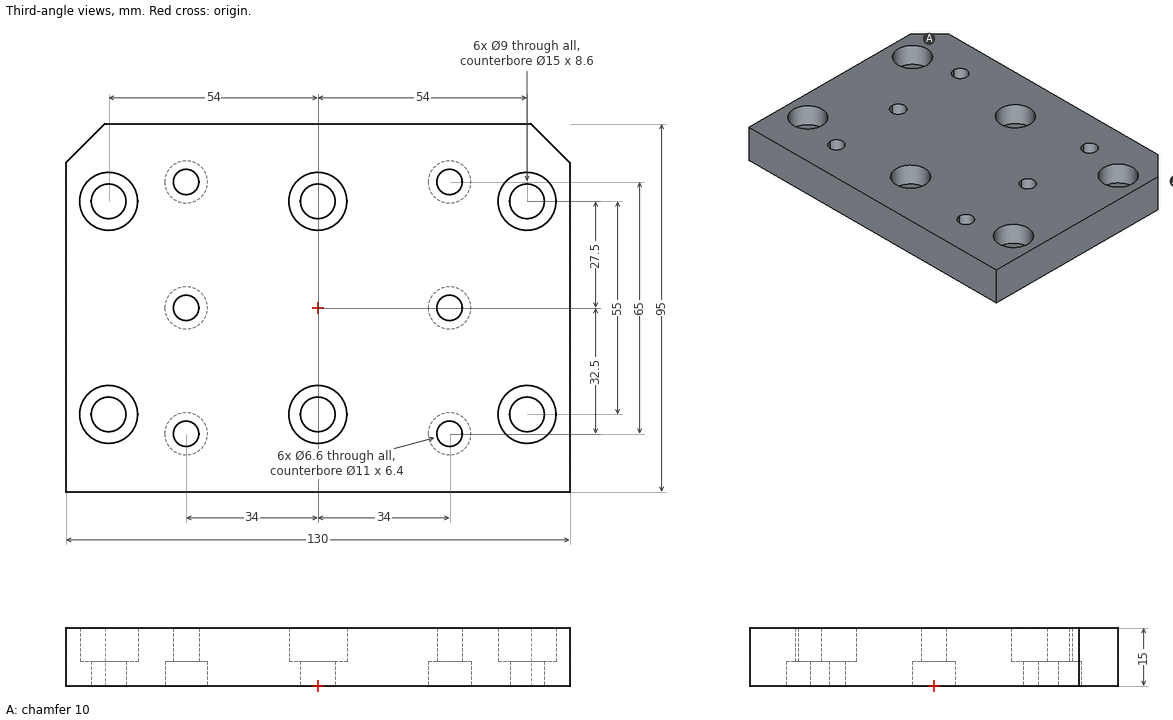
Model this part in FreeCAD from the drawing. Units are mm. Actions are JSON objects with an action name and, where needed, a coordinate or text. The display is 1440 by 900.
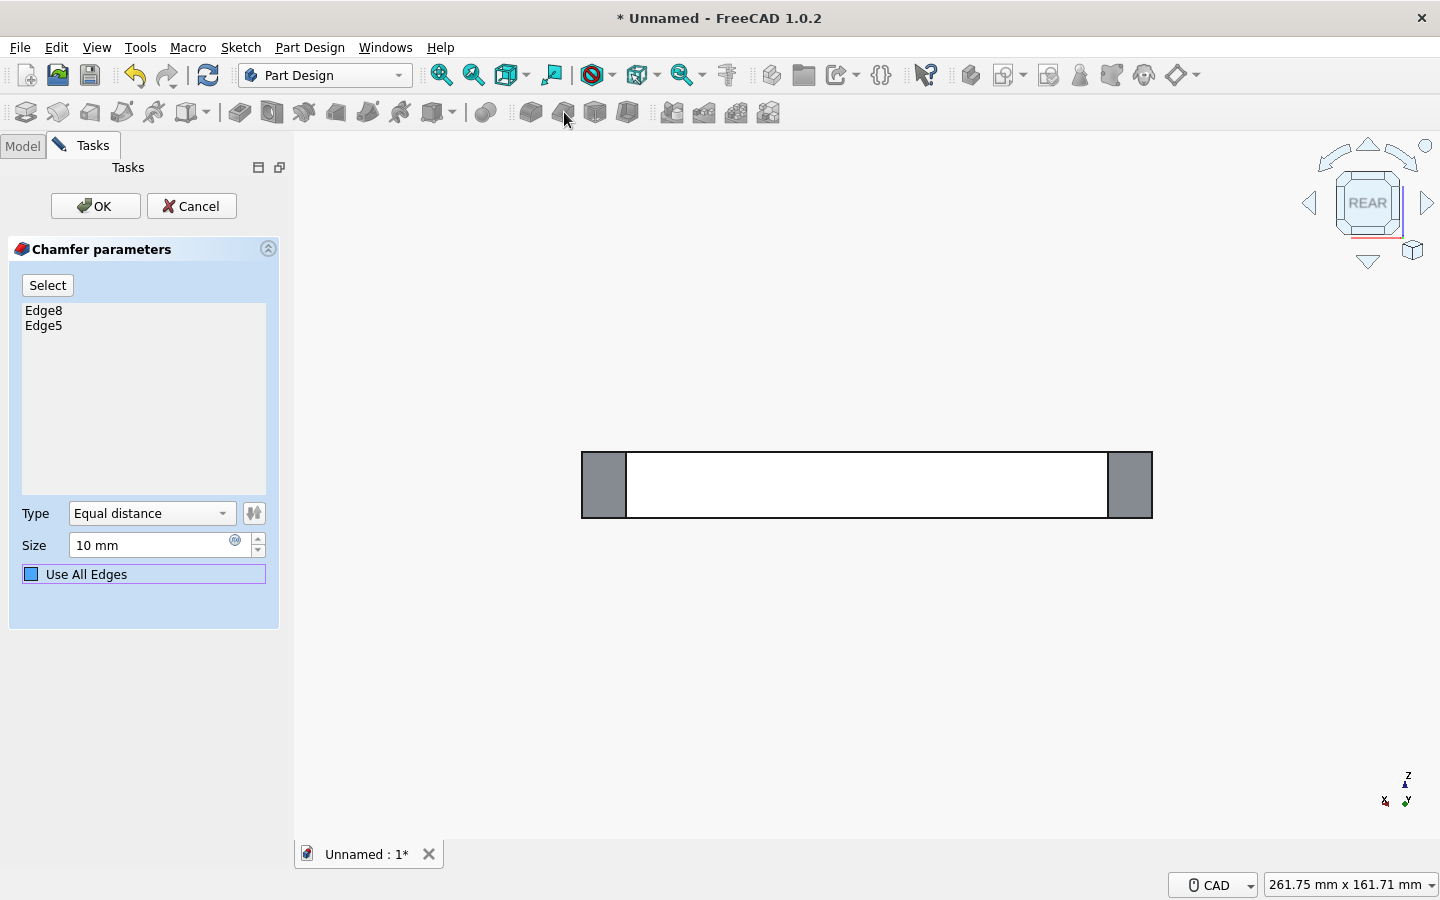
{"action": "left_click", "coordinate": [96, 206]}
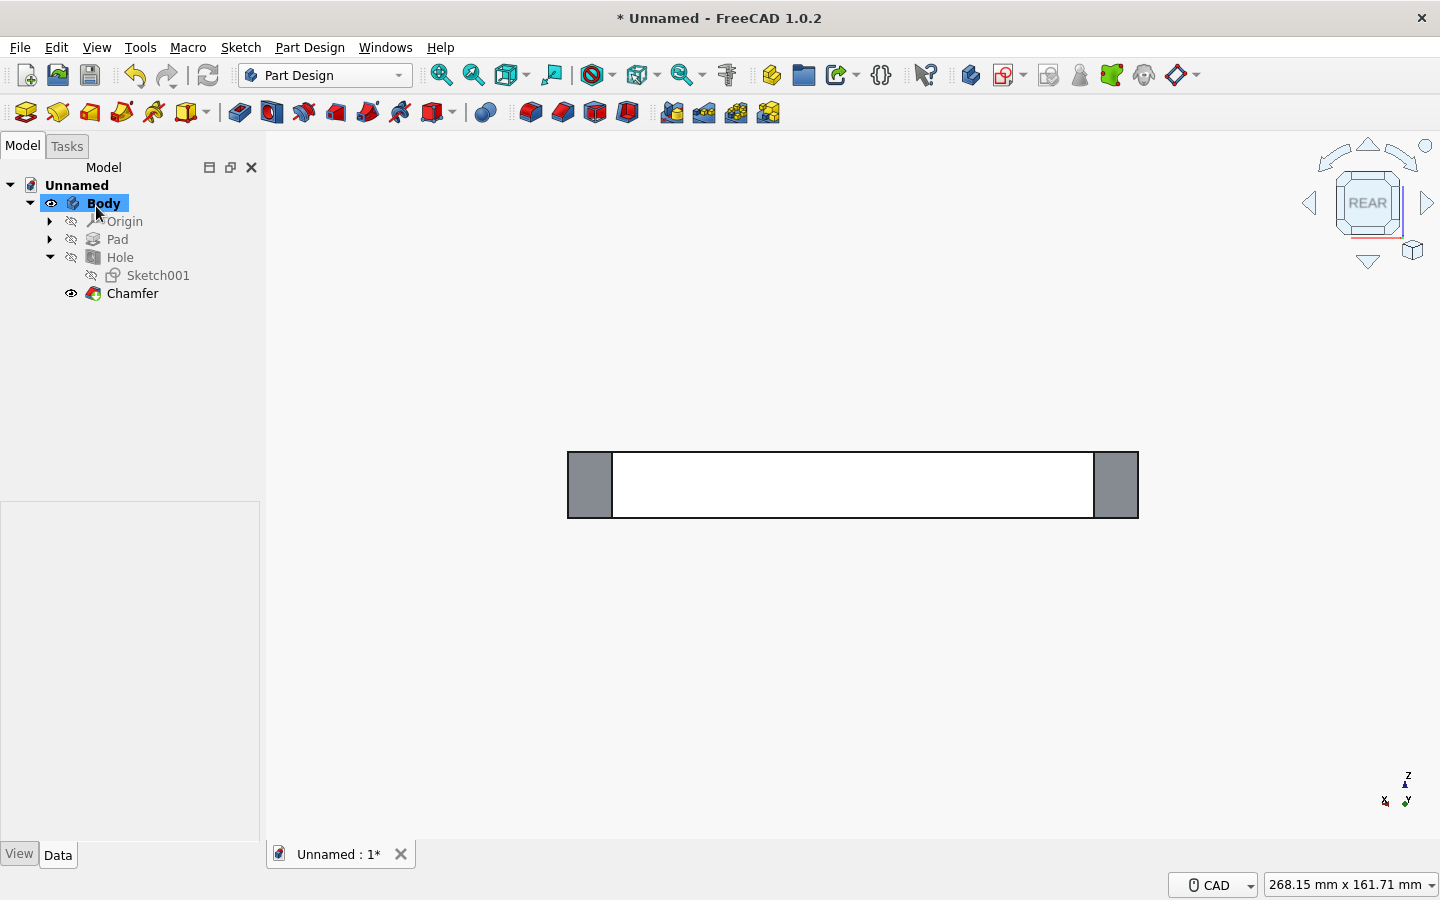
{"action": "left_click", "coordinate": [1004, 76]}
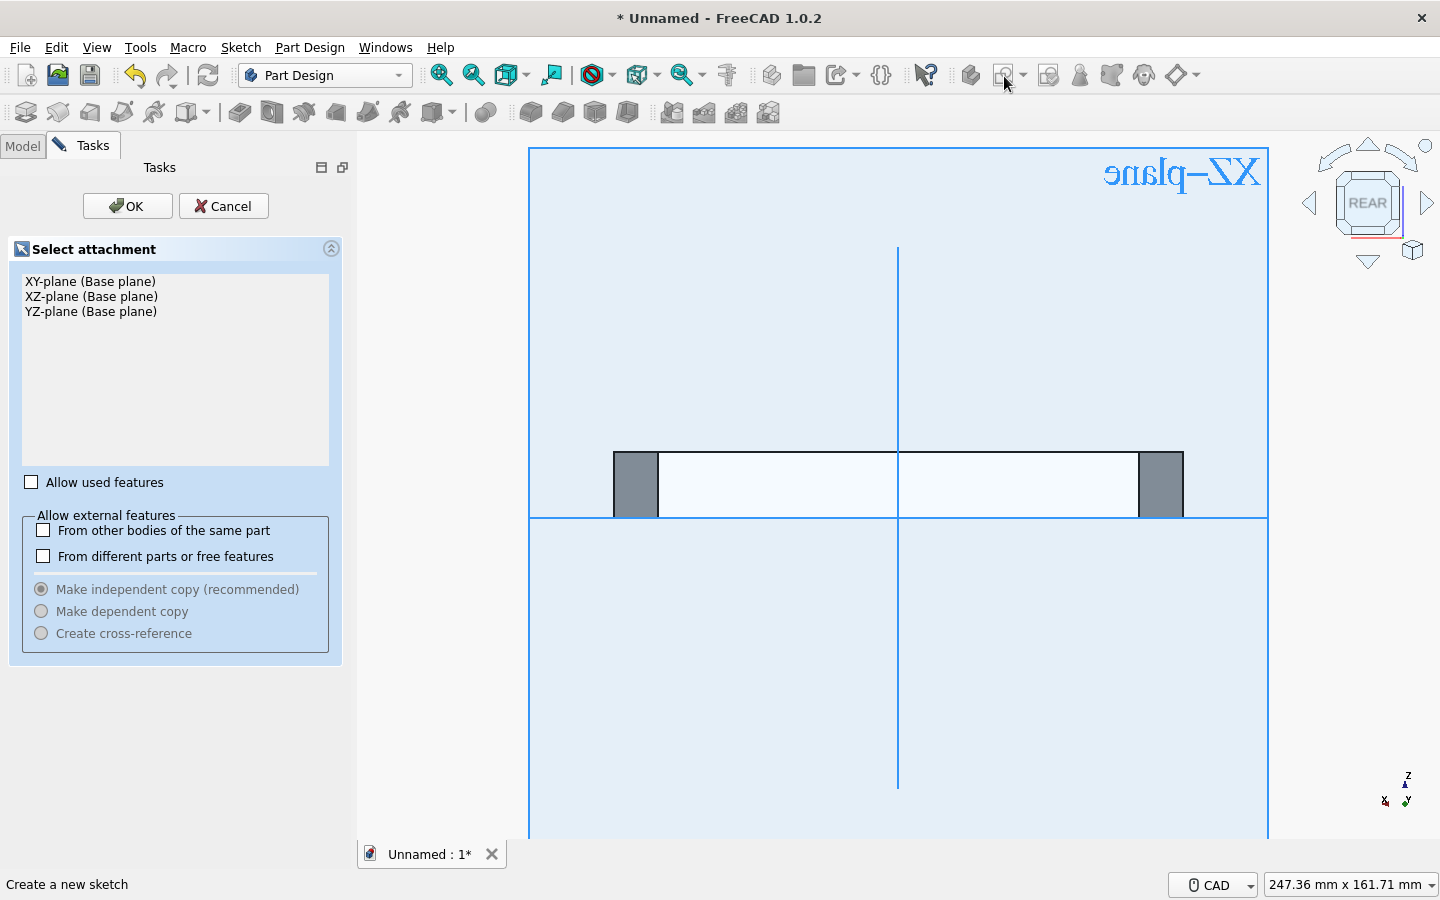
{"action": "left_click", "coordinate": [82, 282]}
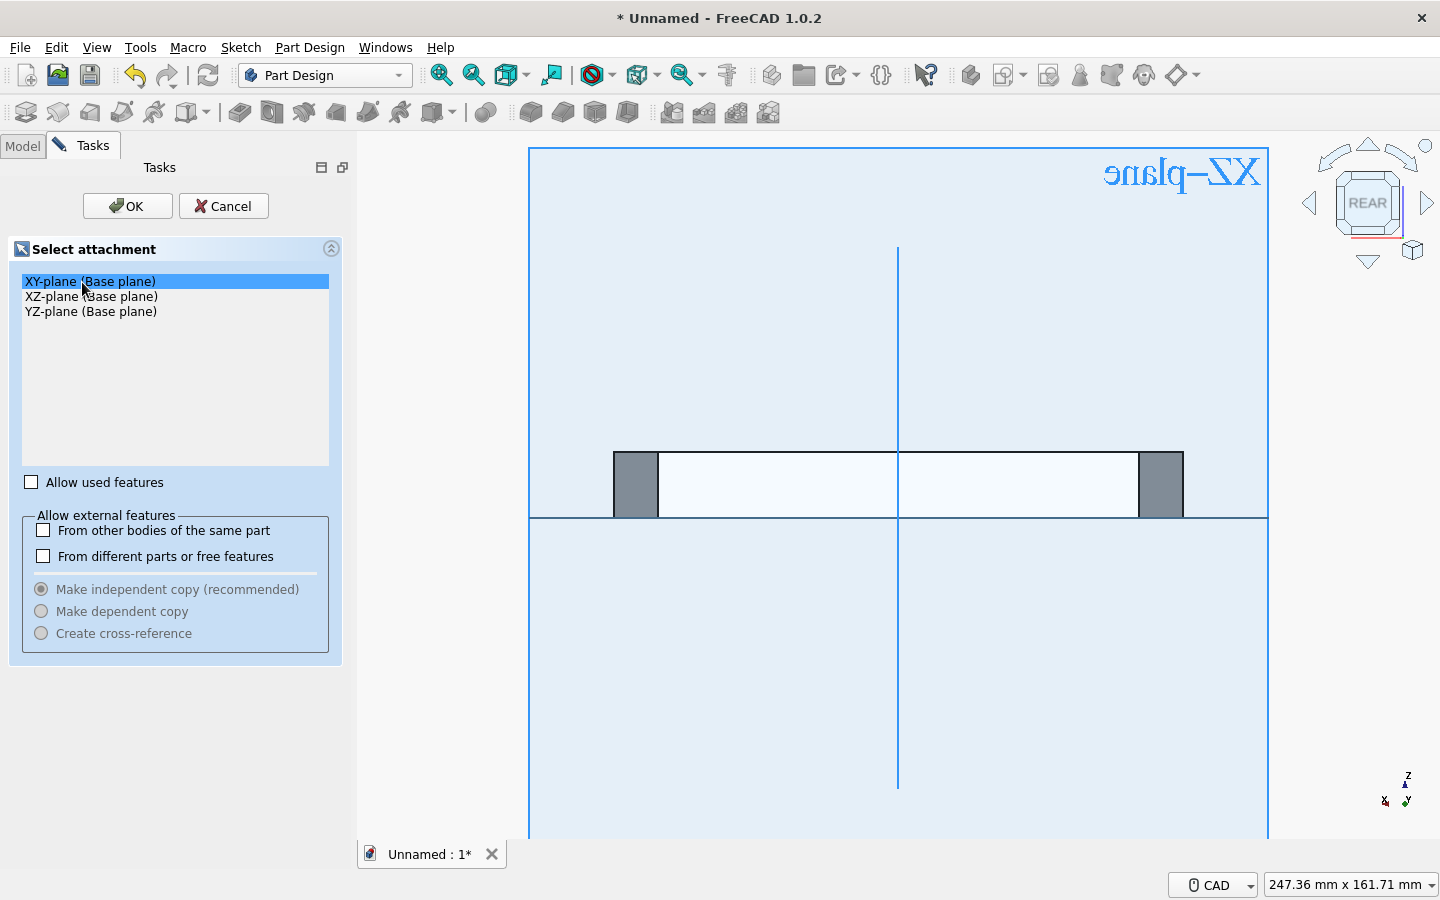
{"action": "left_click", "coordinate": [128, 206]}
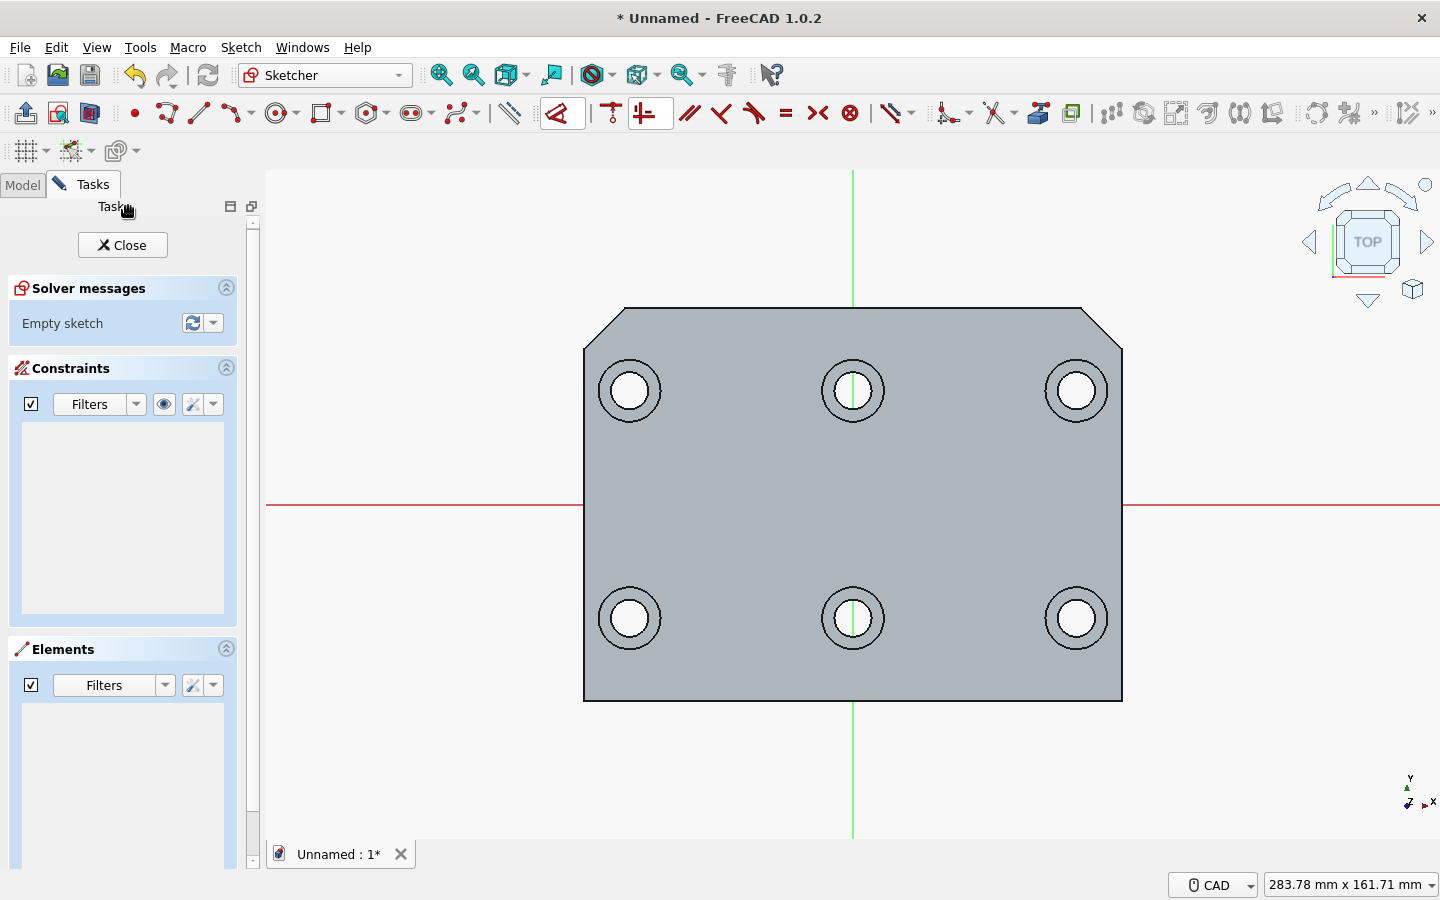
{"action": "left_click", "coordinate": [90, 114]}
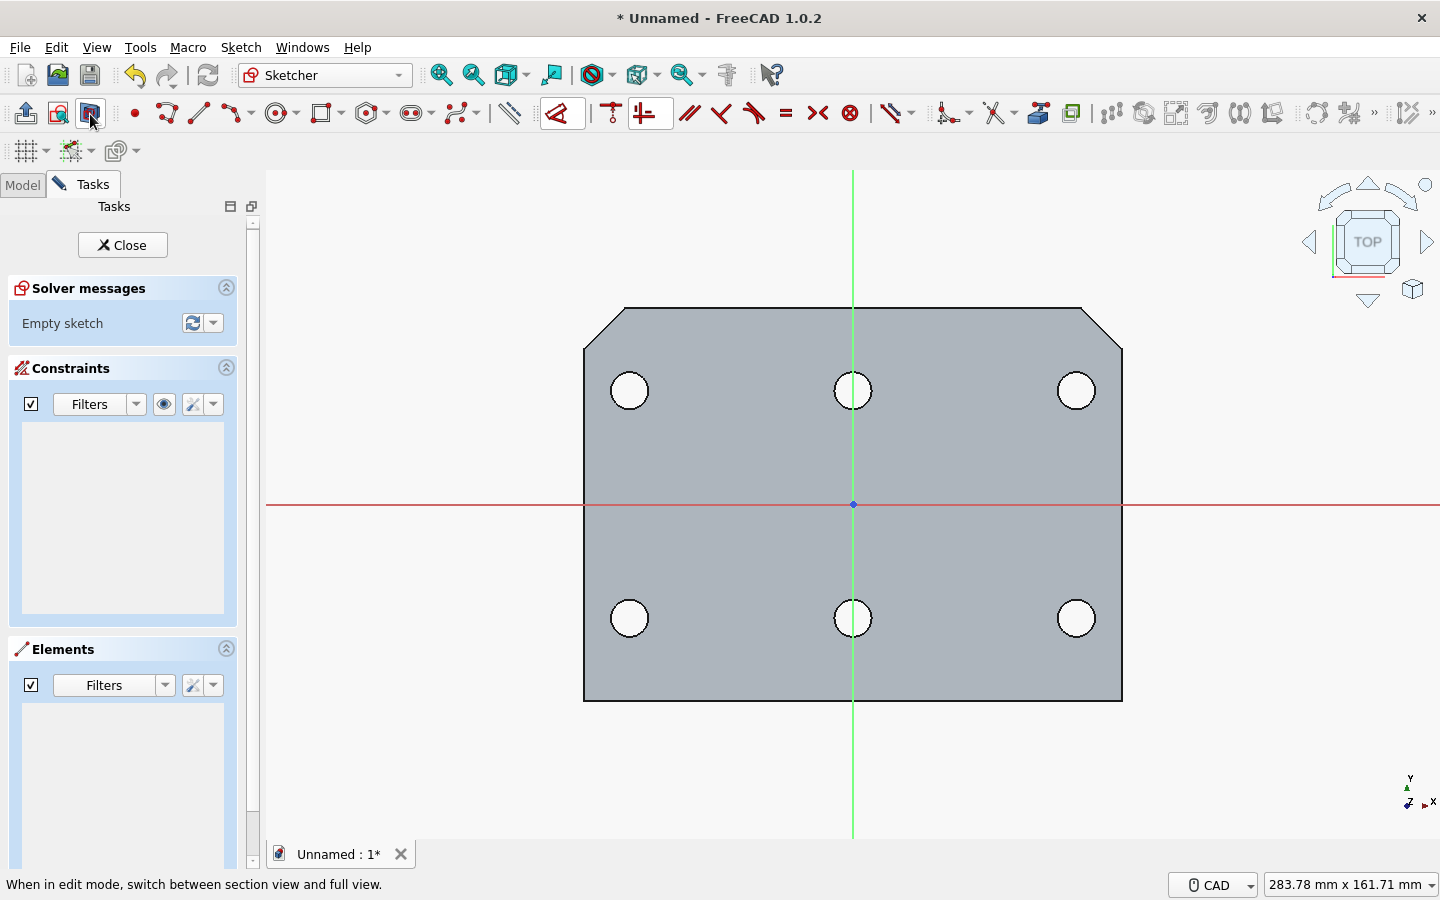
{"action": "scroll", "coordinate": [992, 505], "scroll_direction": "up", "scroll_amount": 2}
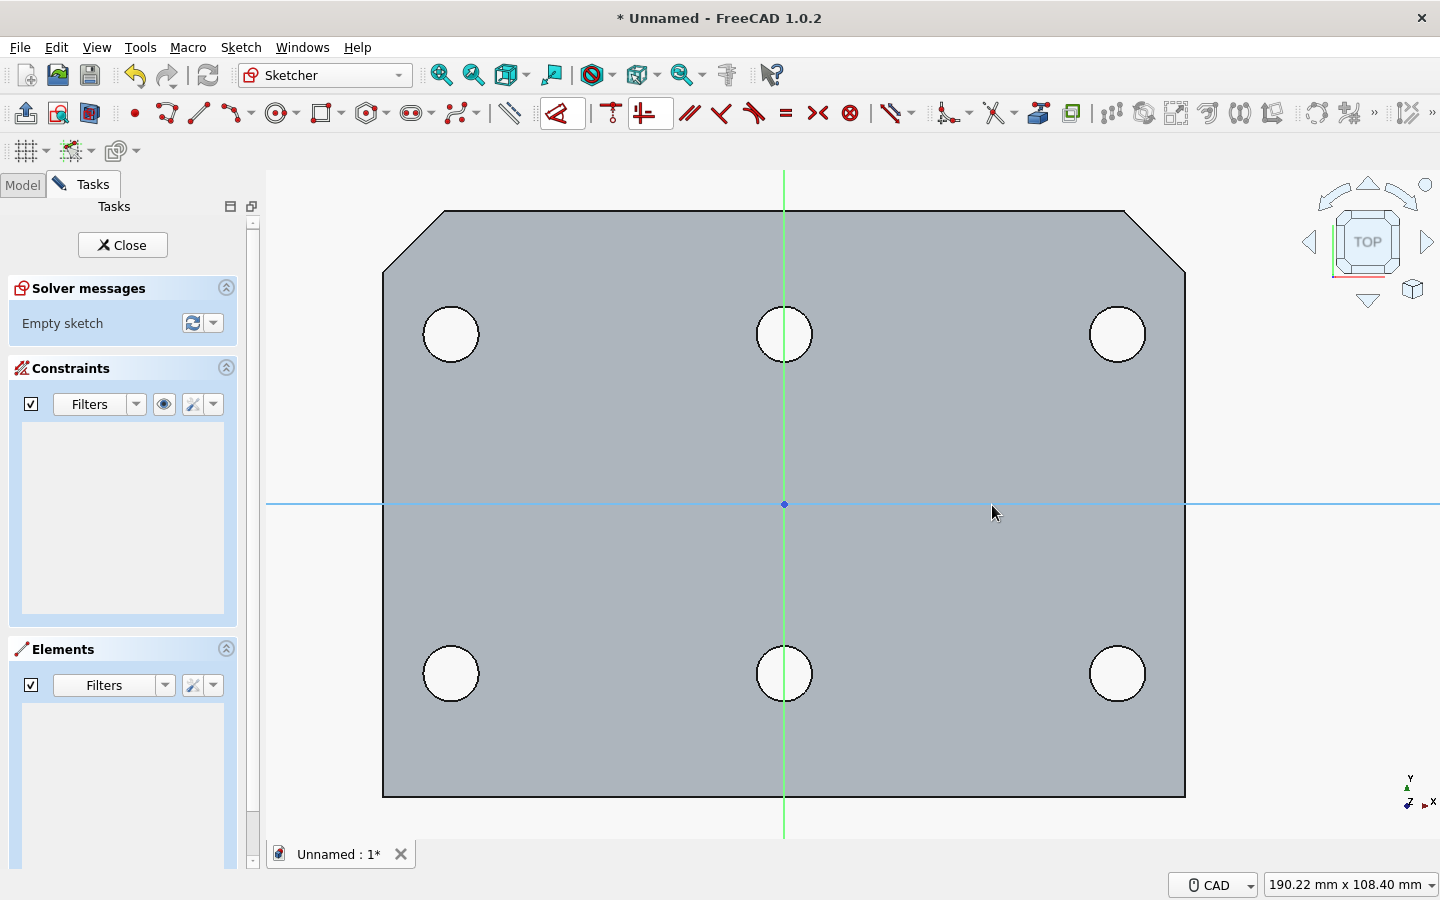
{"action": "key", "text": "g c"}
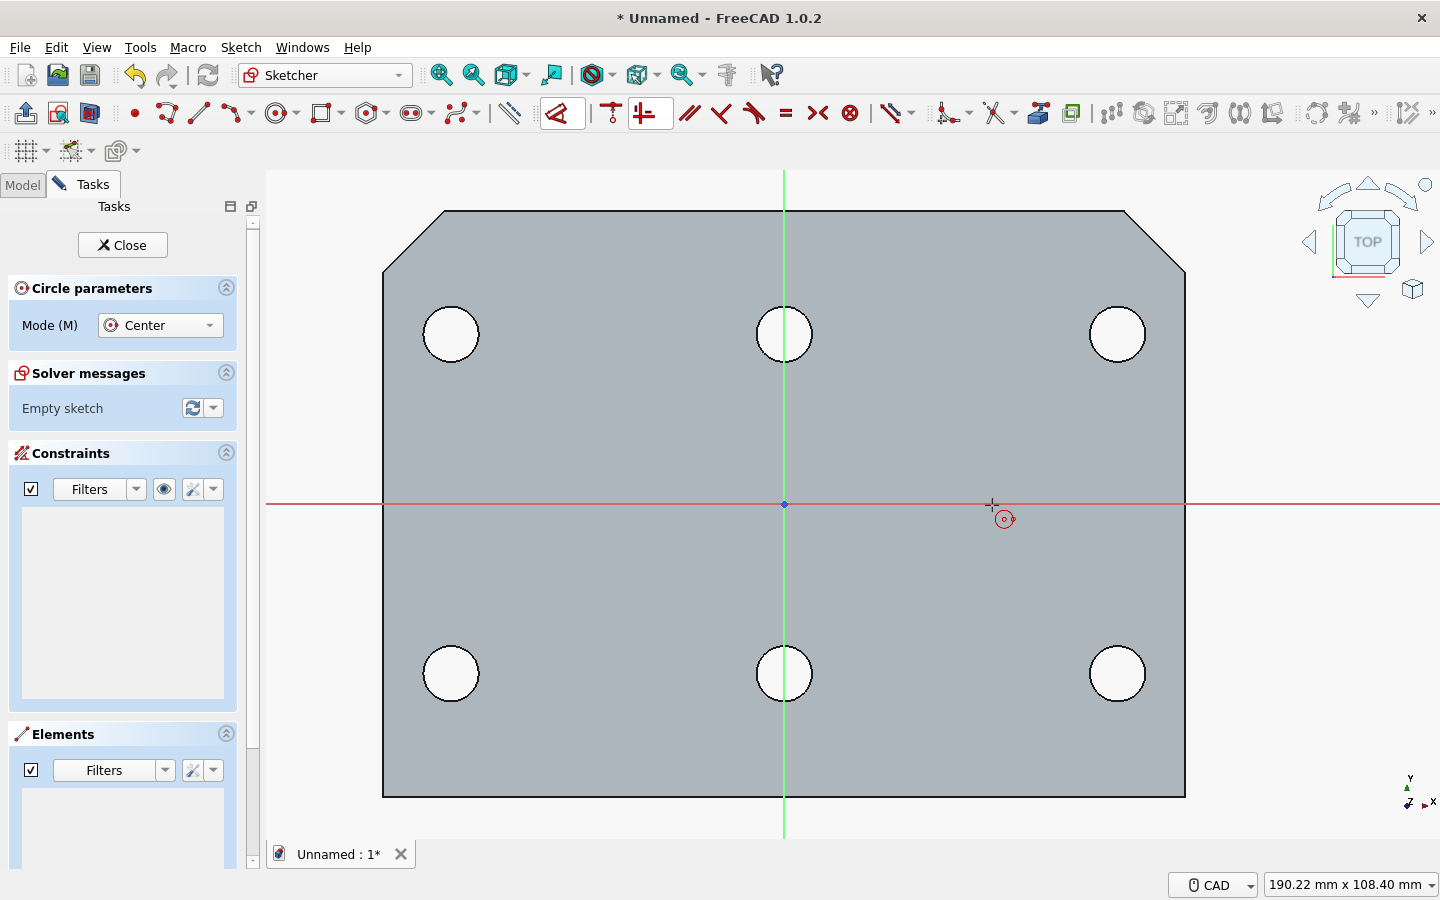
{"action": "left_click", "coordinate": [994, 705]}
{"action": "mouse_move", "coordinate": [1009, 690]}